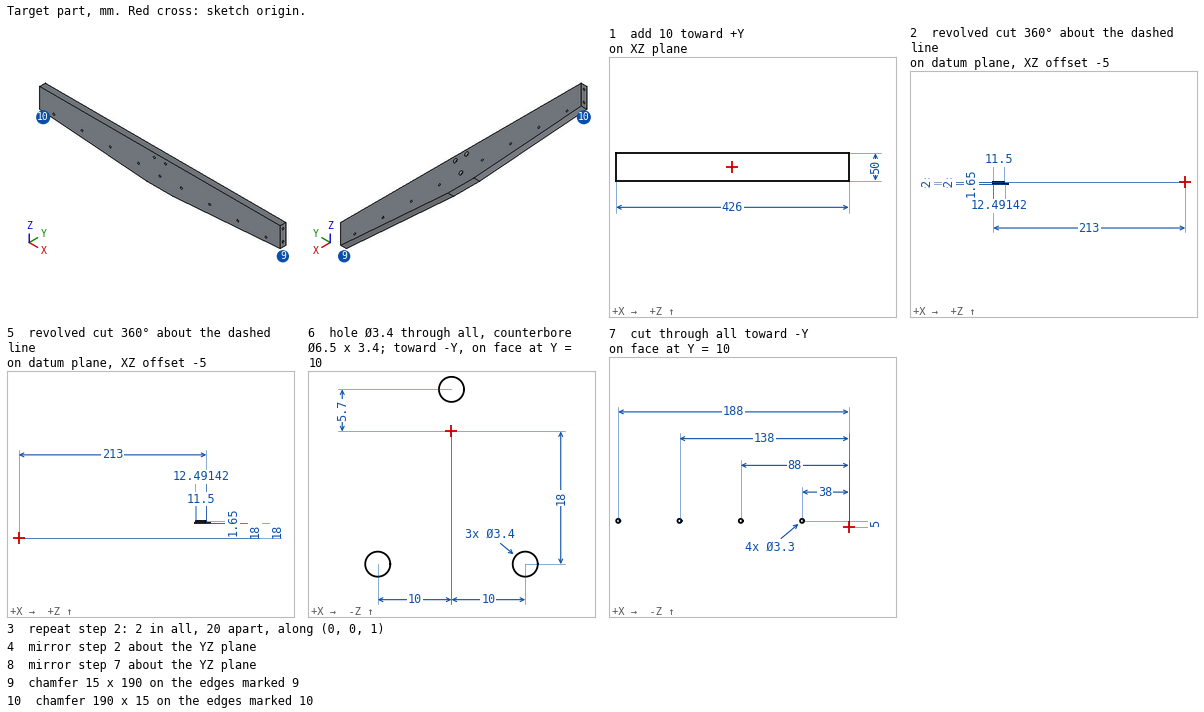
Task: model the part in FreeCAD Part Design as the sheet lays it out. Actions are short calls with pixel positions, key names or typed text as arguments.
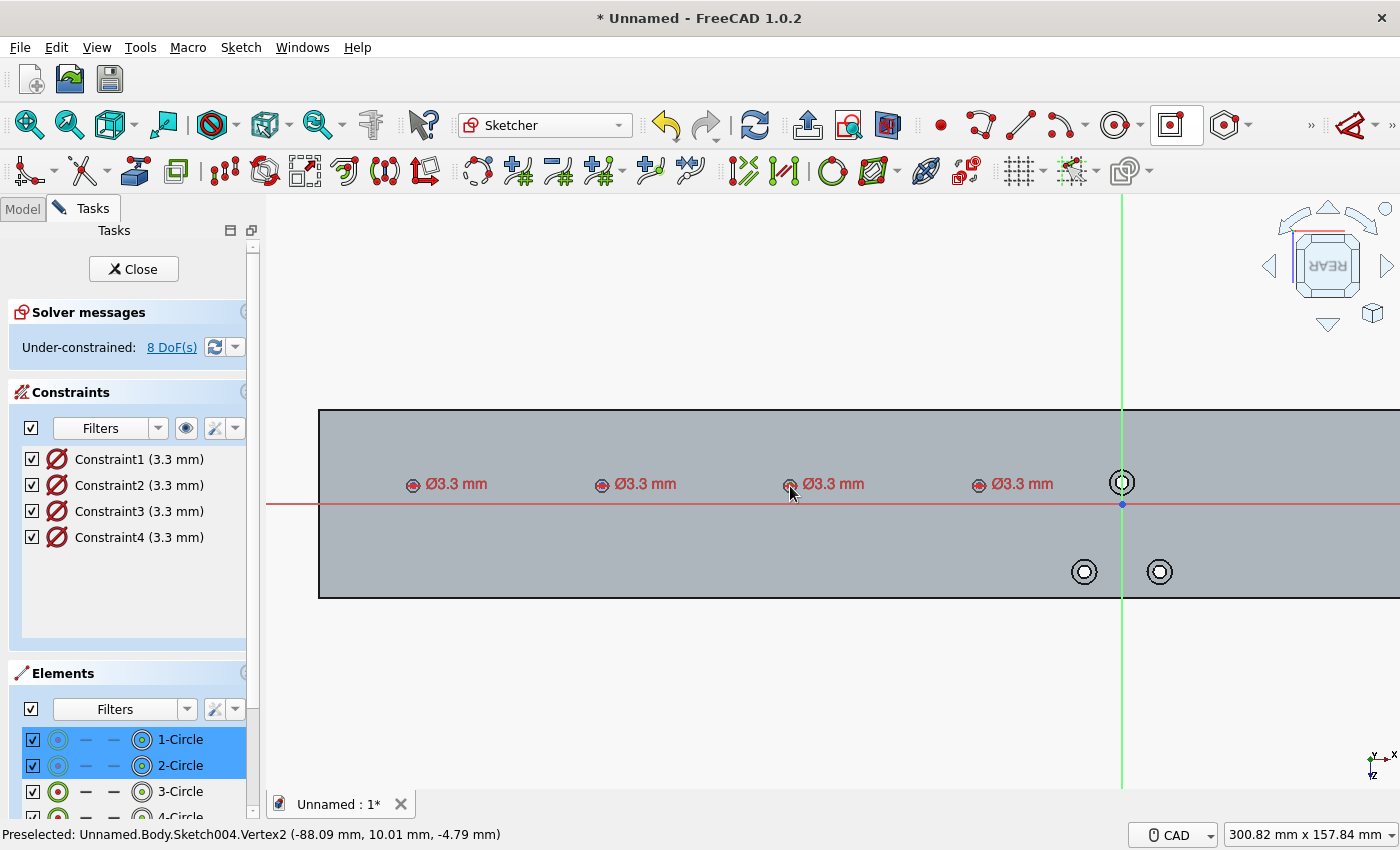
key(h)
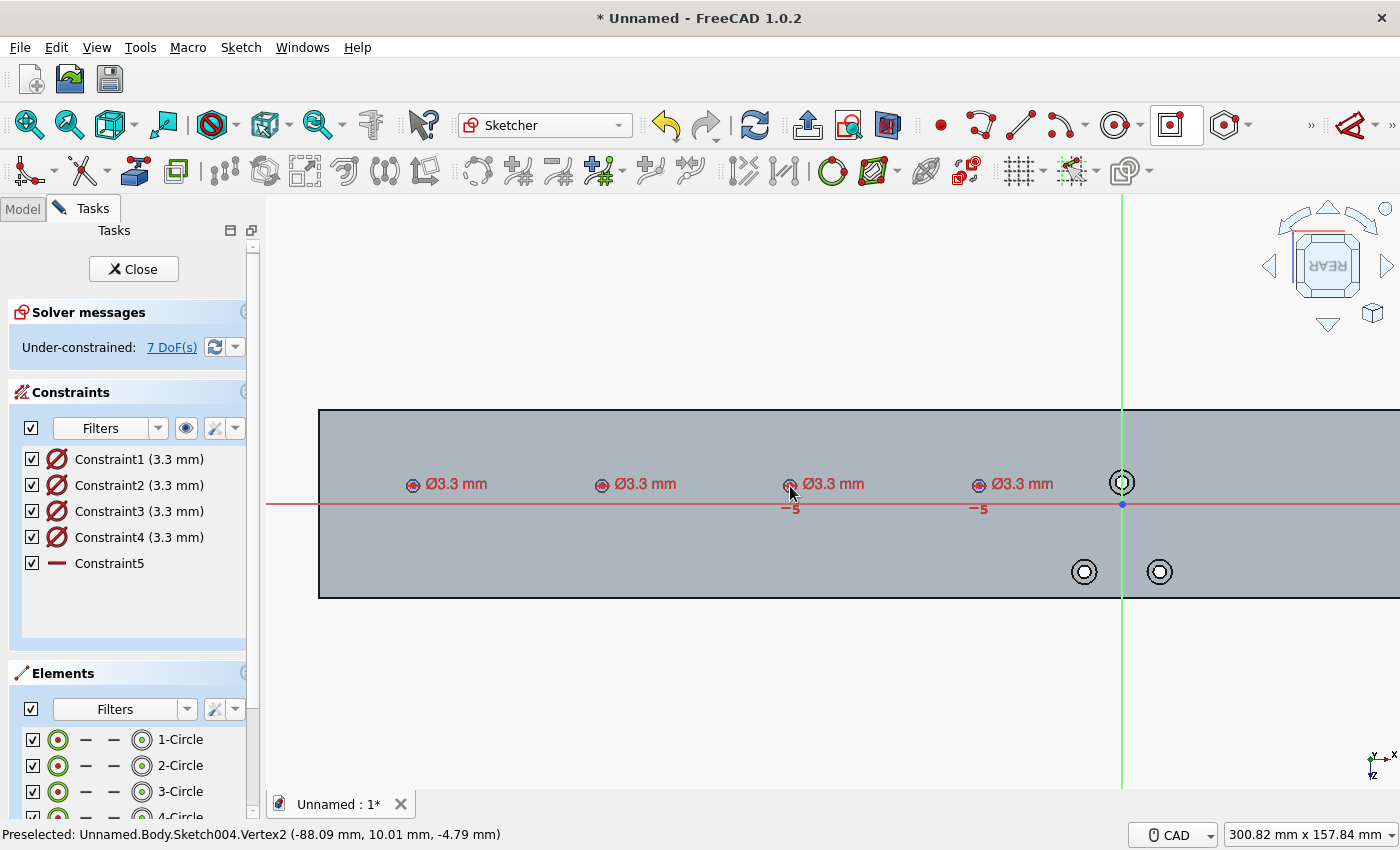
click(790, 486)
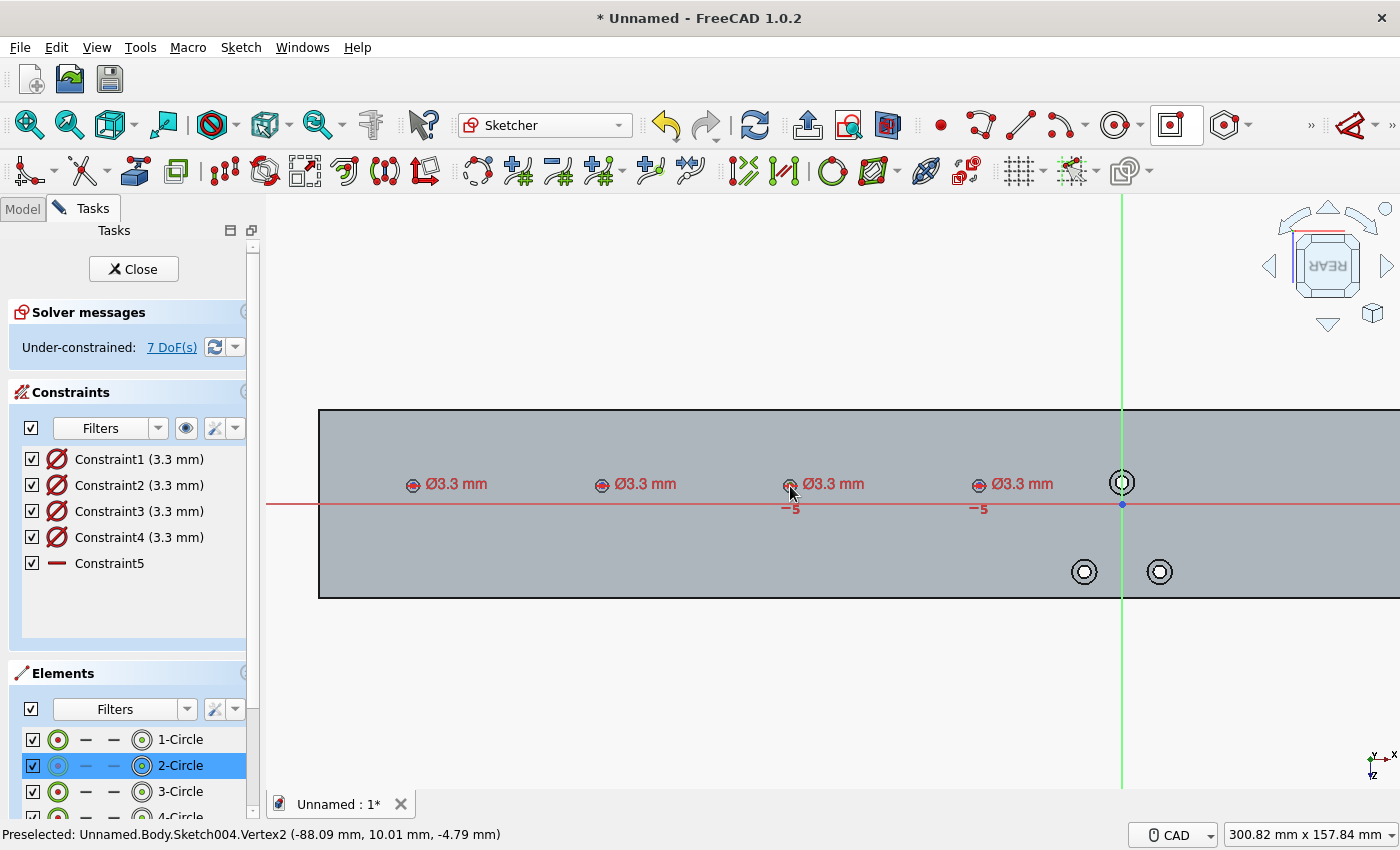
click(602, 486)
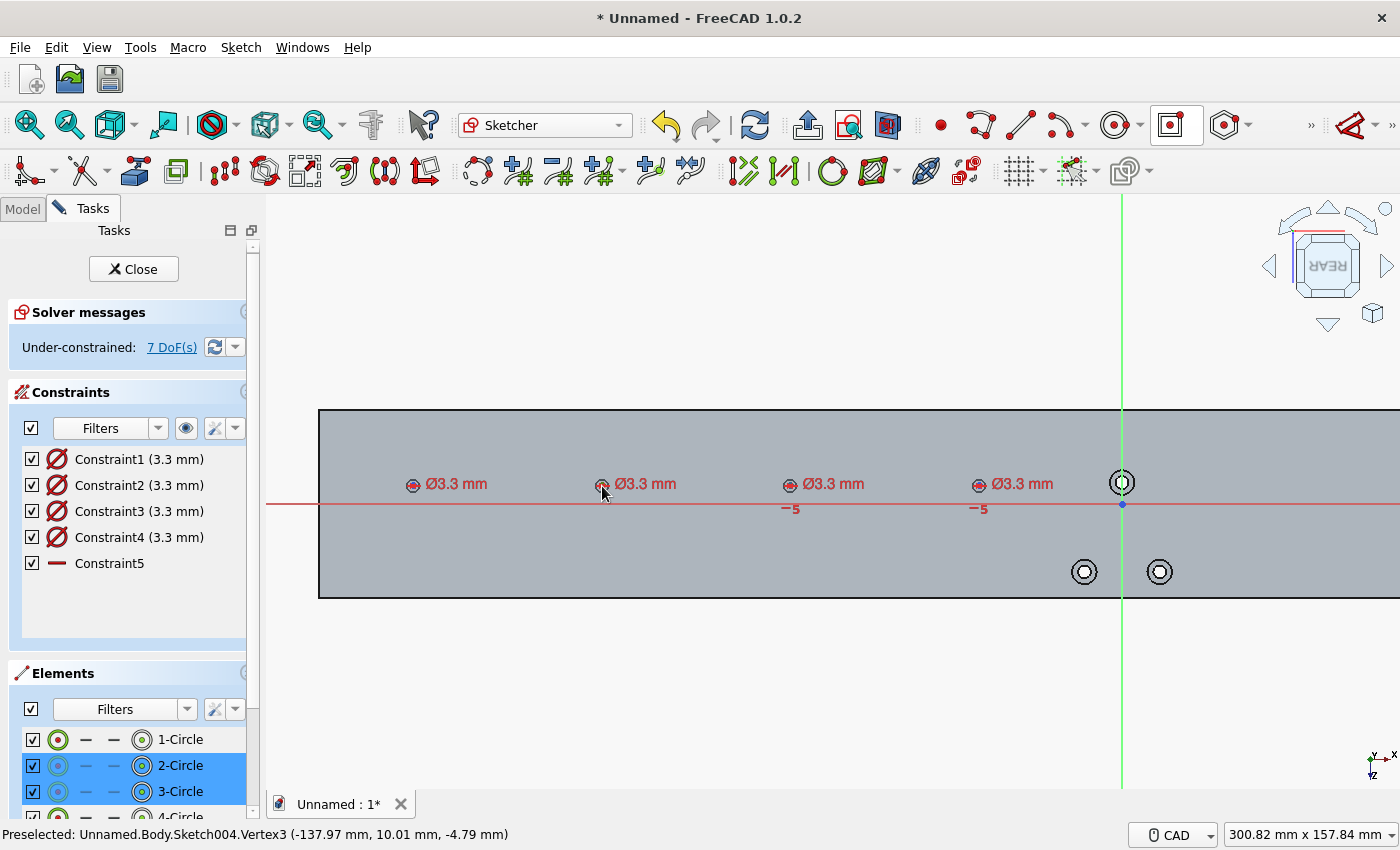
key(h)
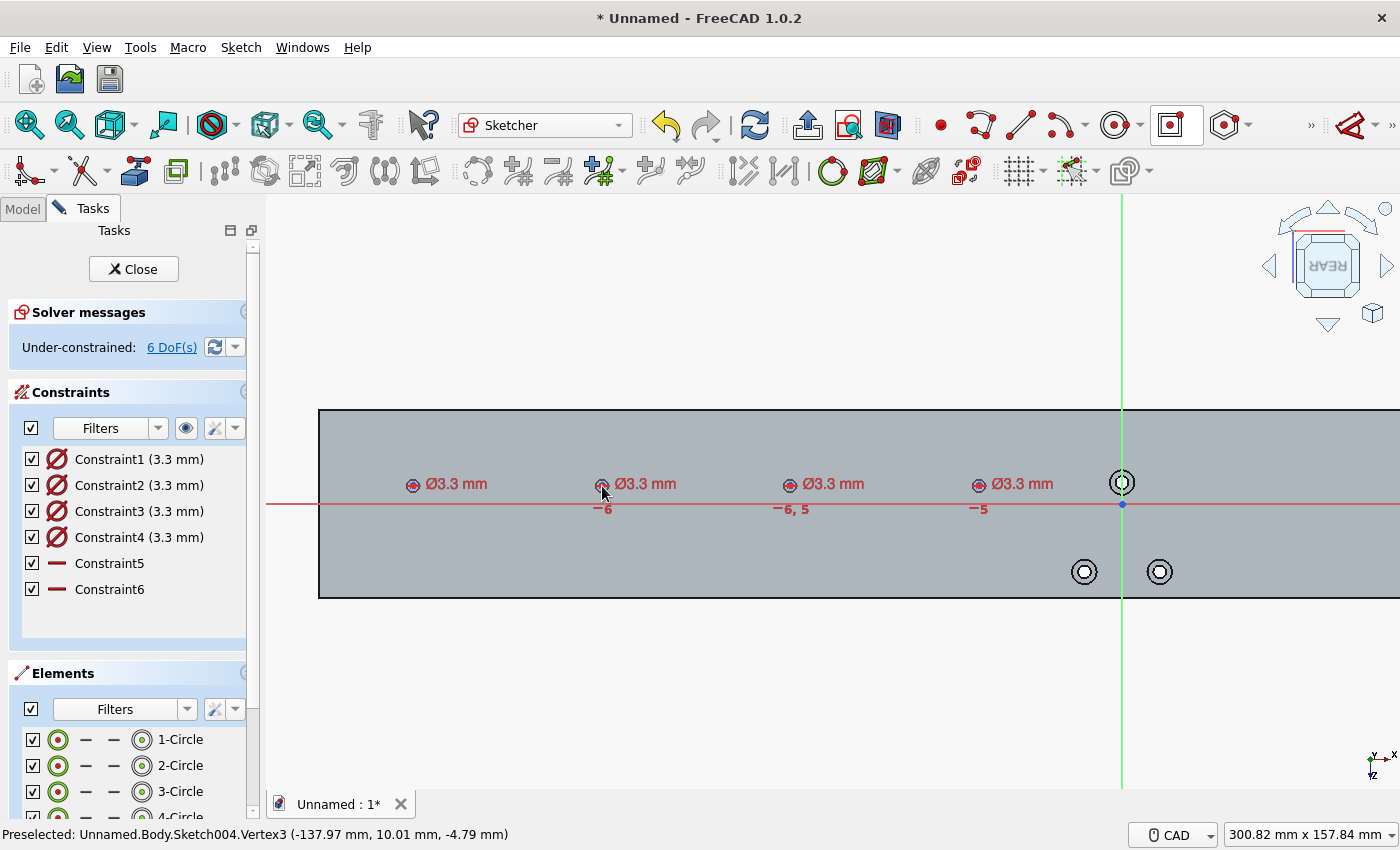
click(602, 486)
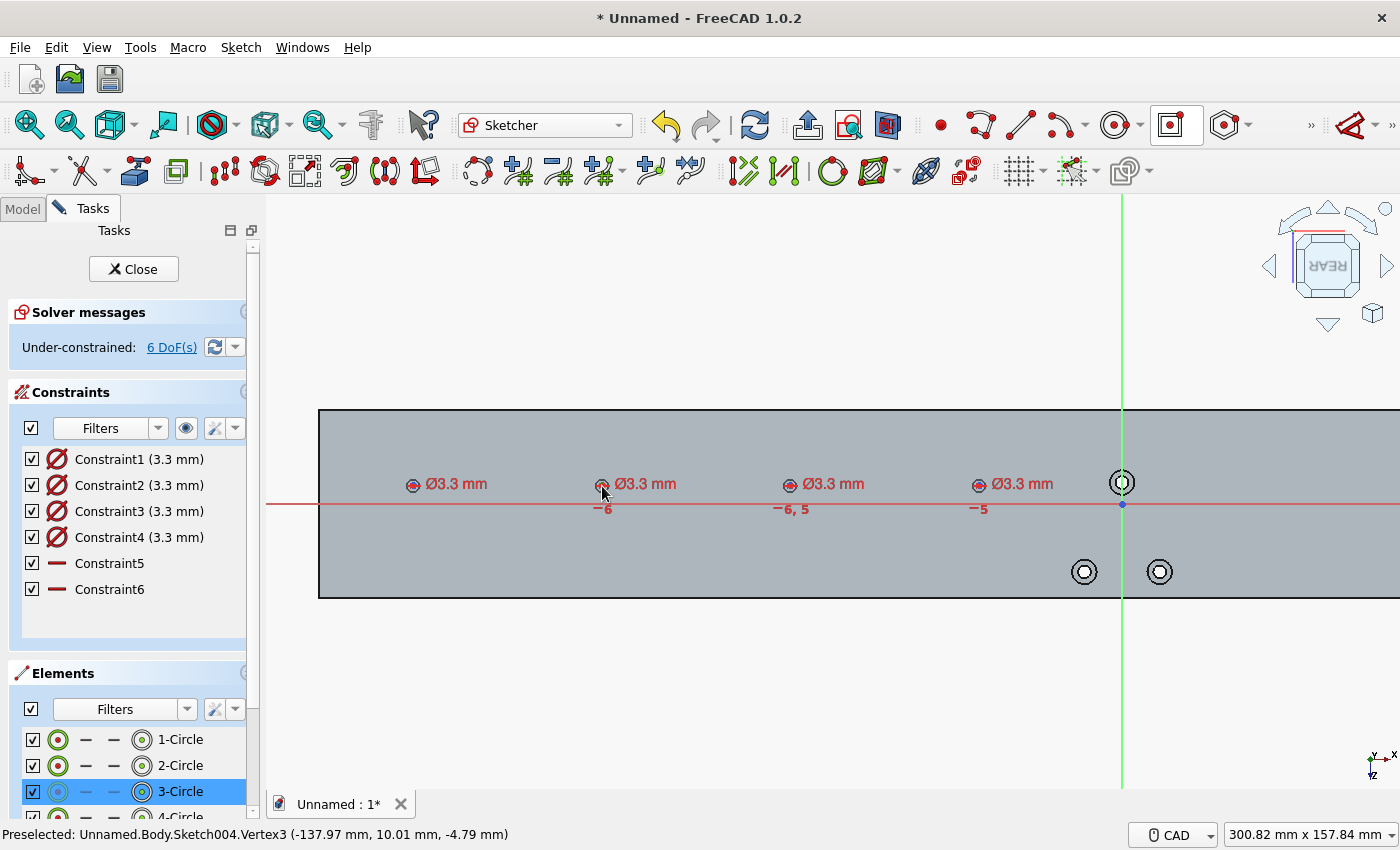
click(413, 486)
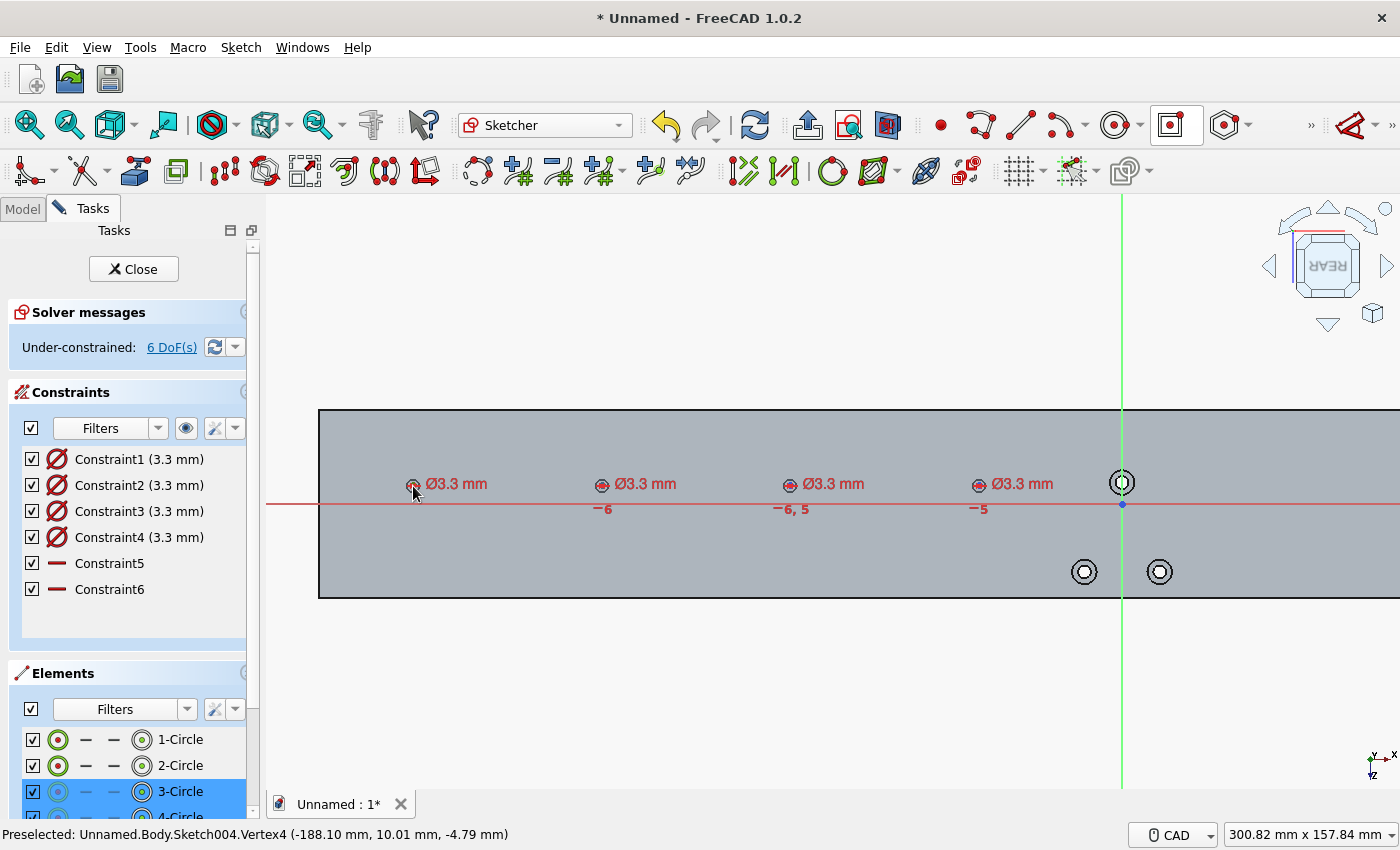
key(h)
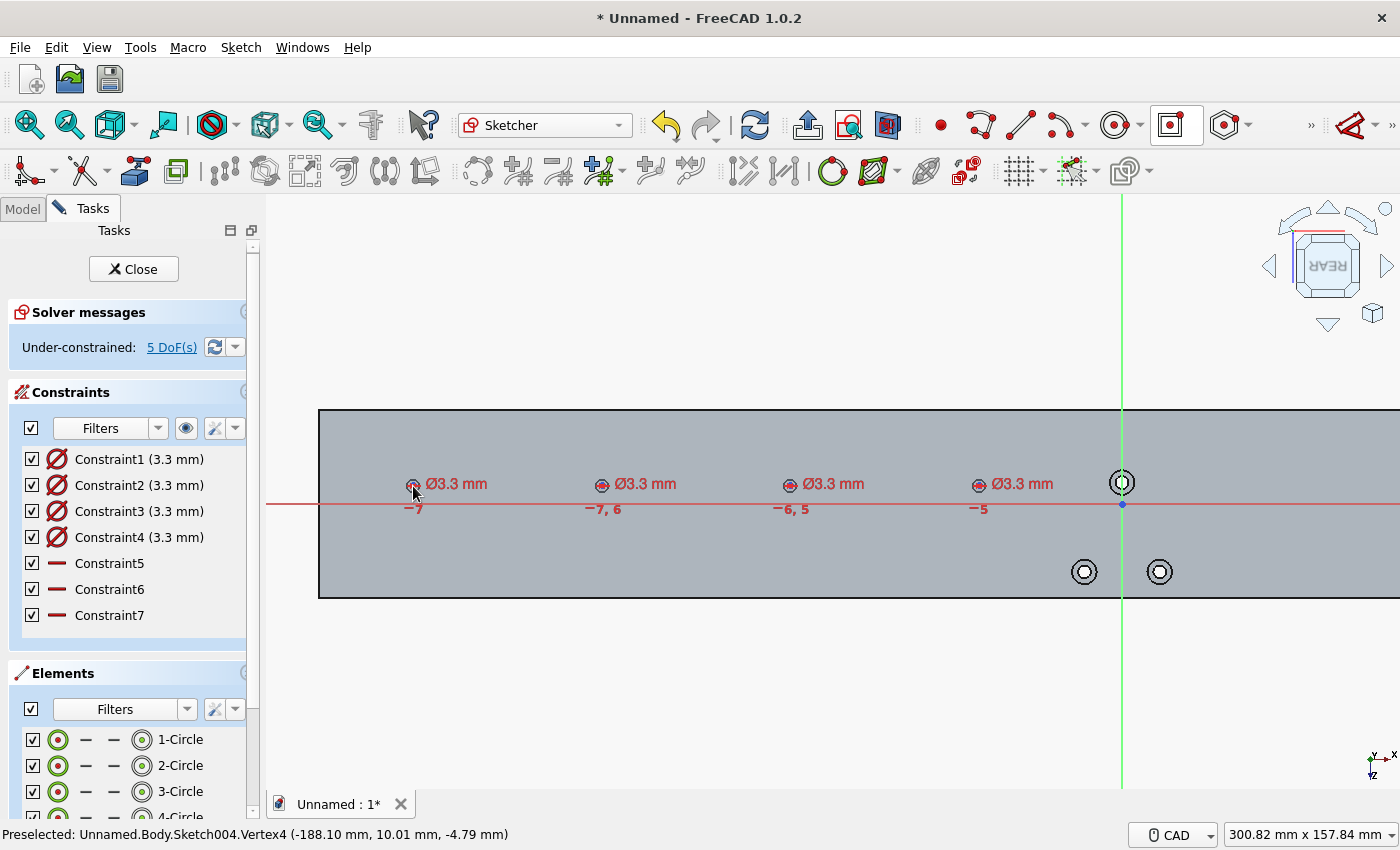
click(1350, 126)